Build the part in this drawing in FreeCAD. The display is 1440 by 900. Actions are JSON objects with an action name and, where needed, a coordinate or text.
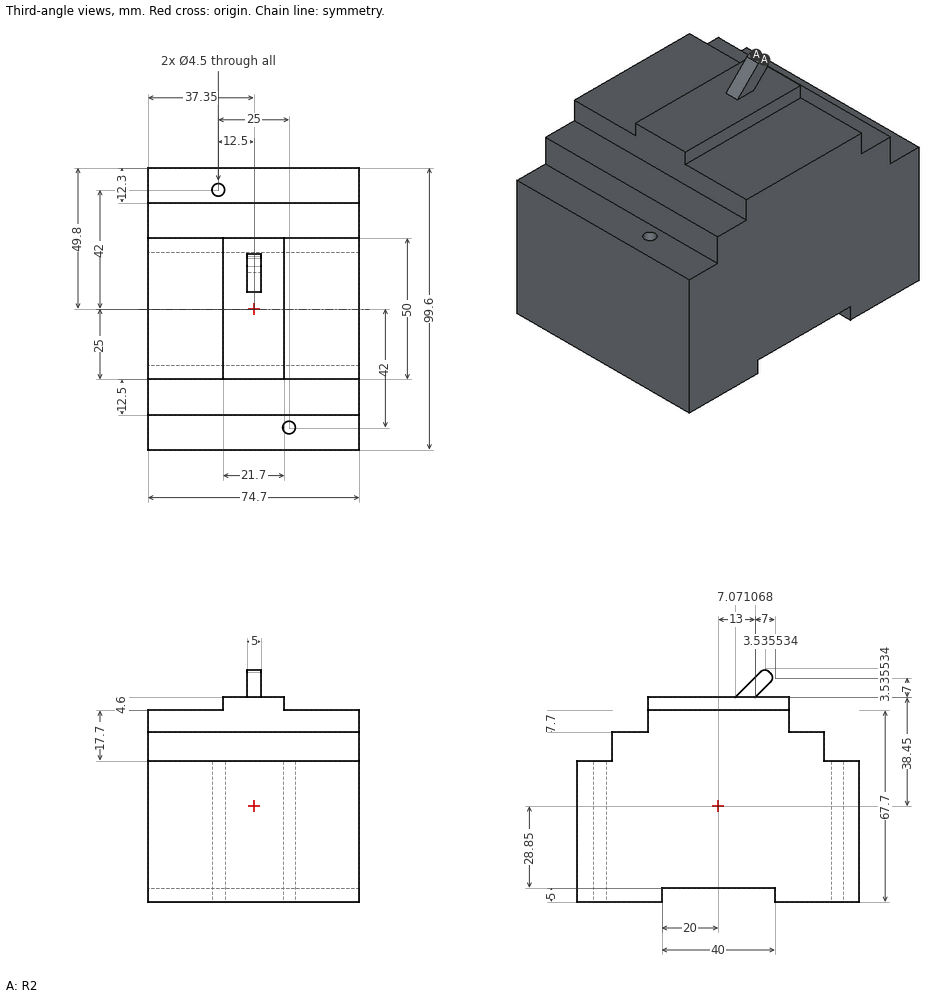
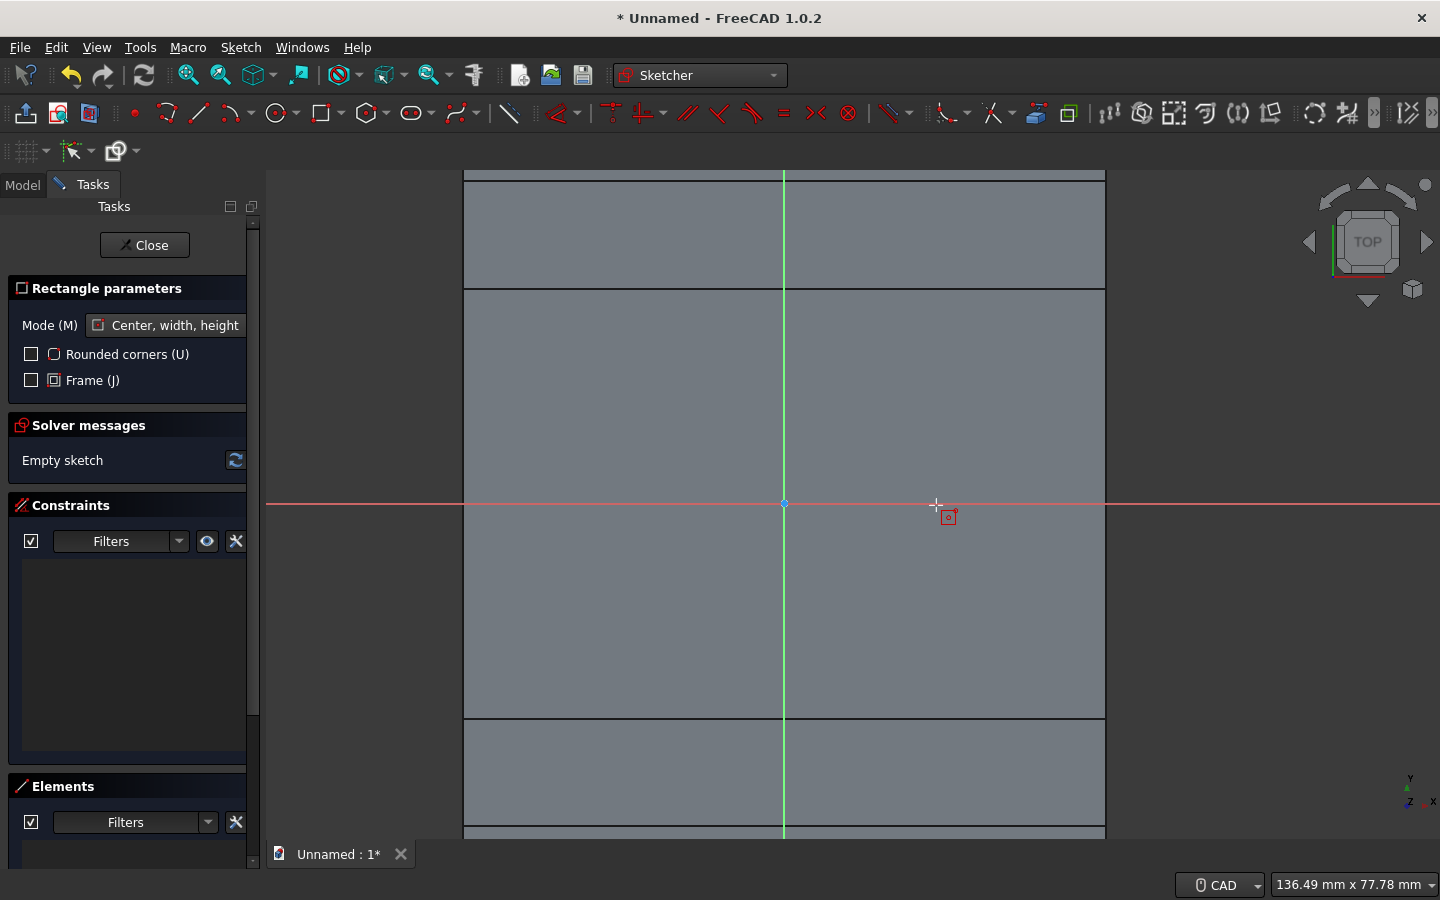
{"action": "left_click", "coordinate": [784, 504]}
{"action": "left_click", "coordinate": [878, 289]}
{"action": "key", "text": "Escape"}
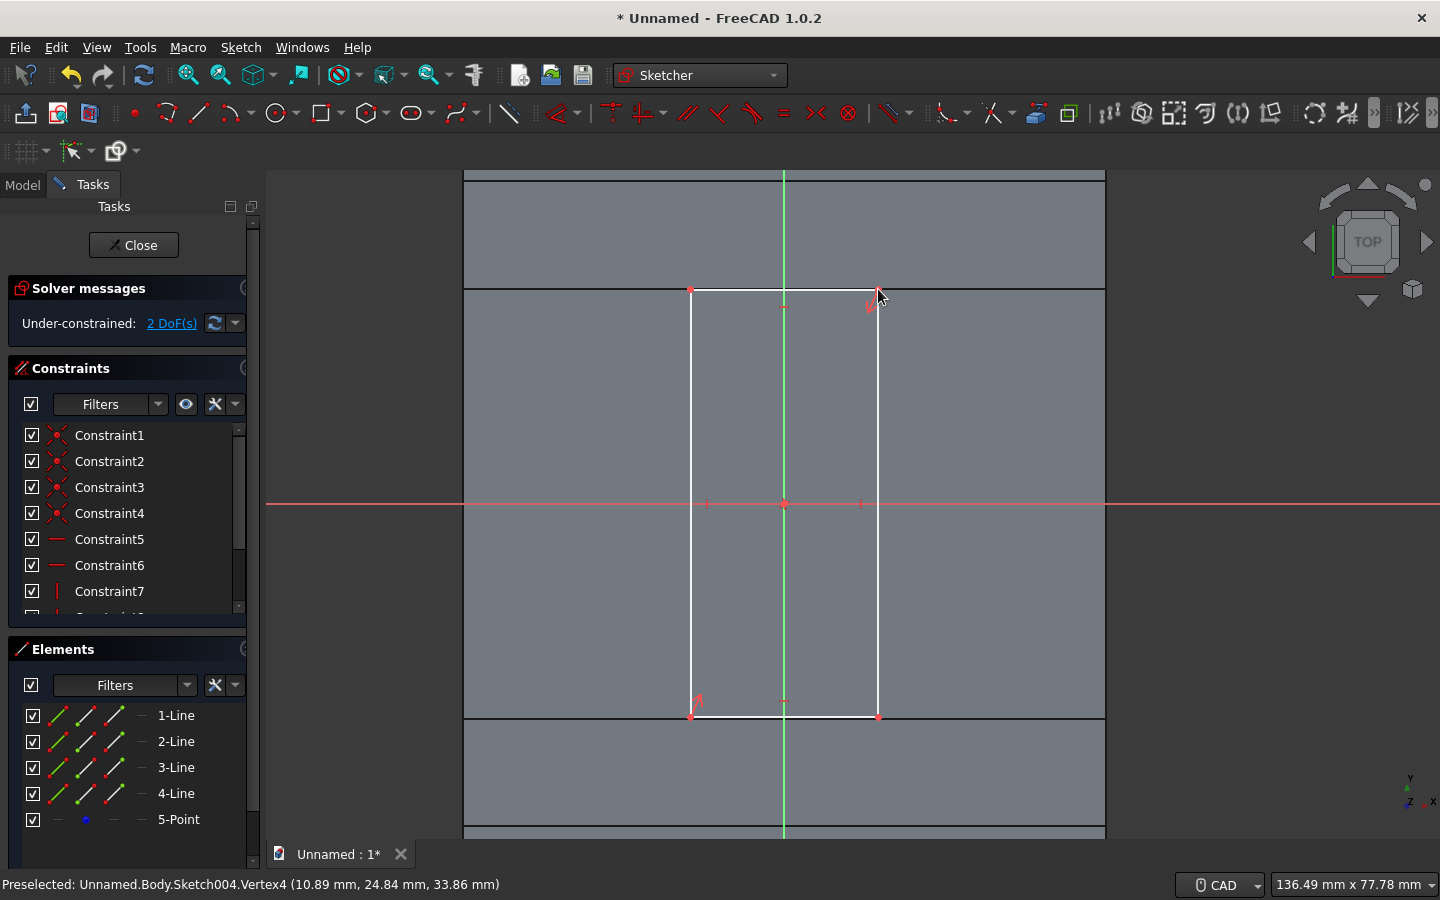
{"action": "left_click", "coordinate": [556, 114]}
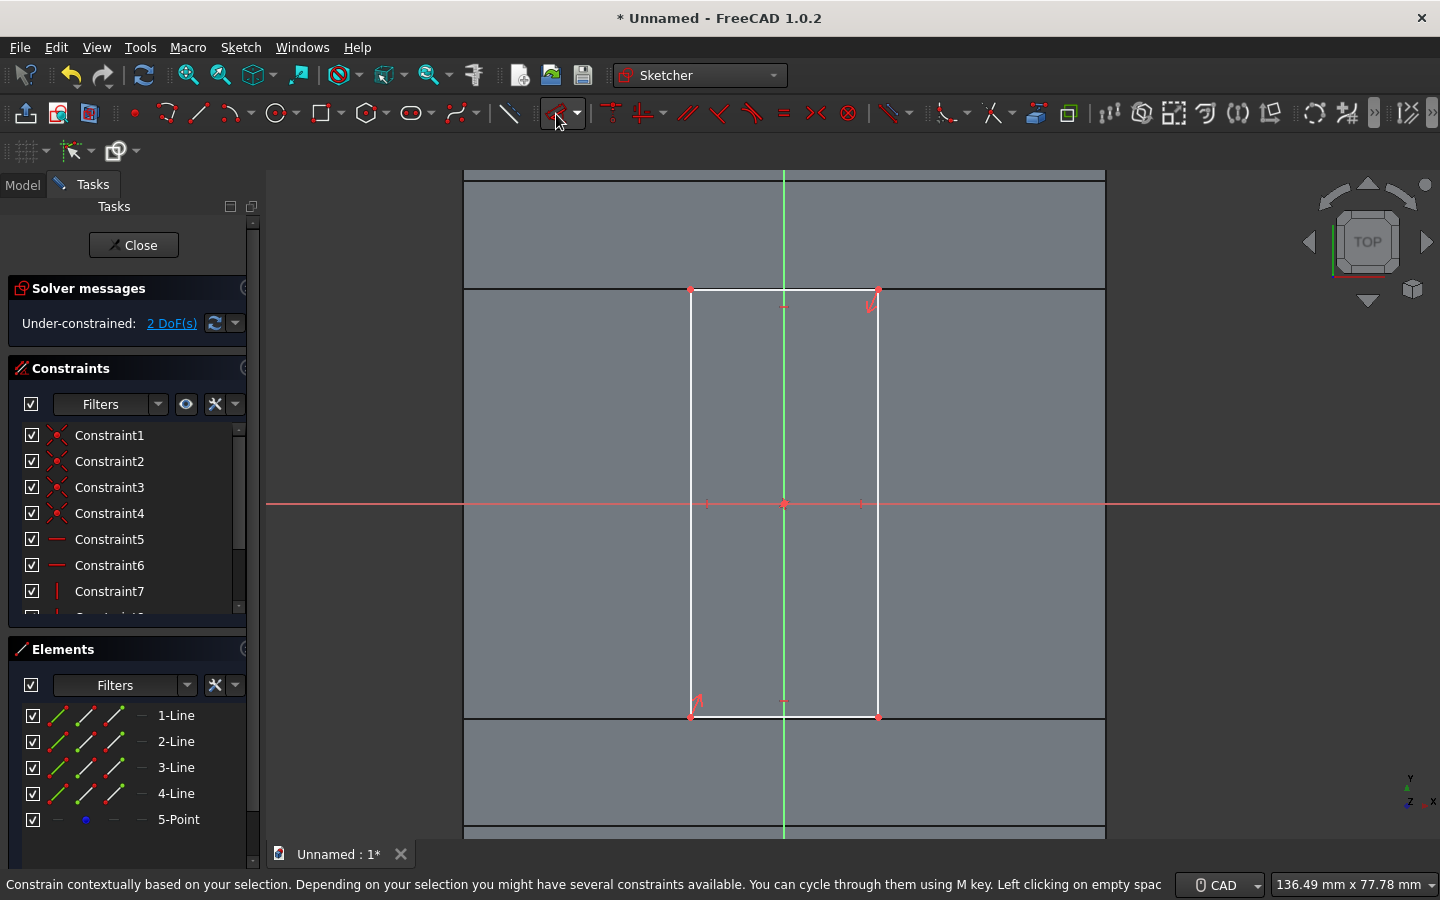
{"action": "left_click", "coordinate": [878, 589]}
{"action": "left_click", "coordinate": [912, 405]}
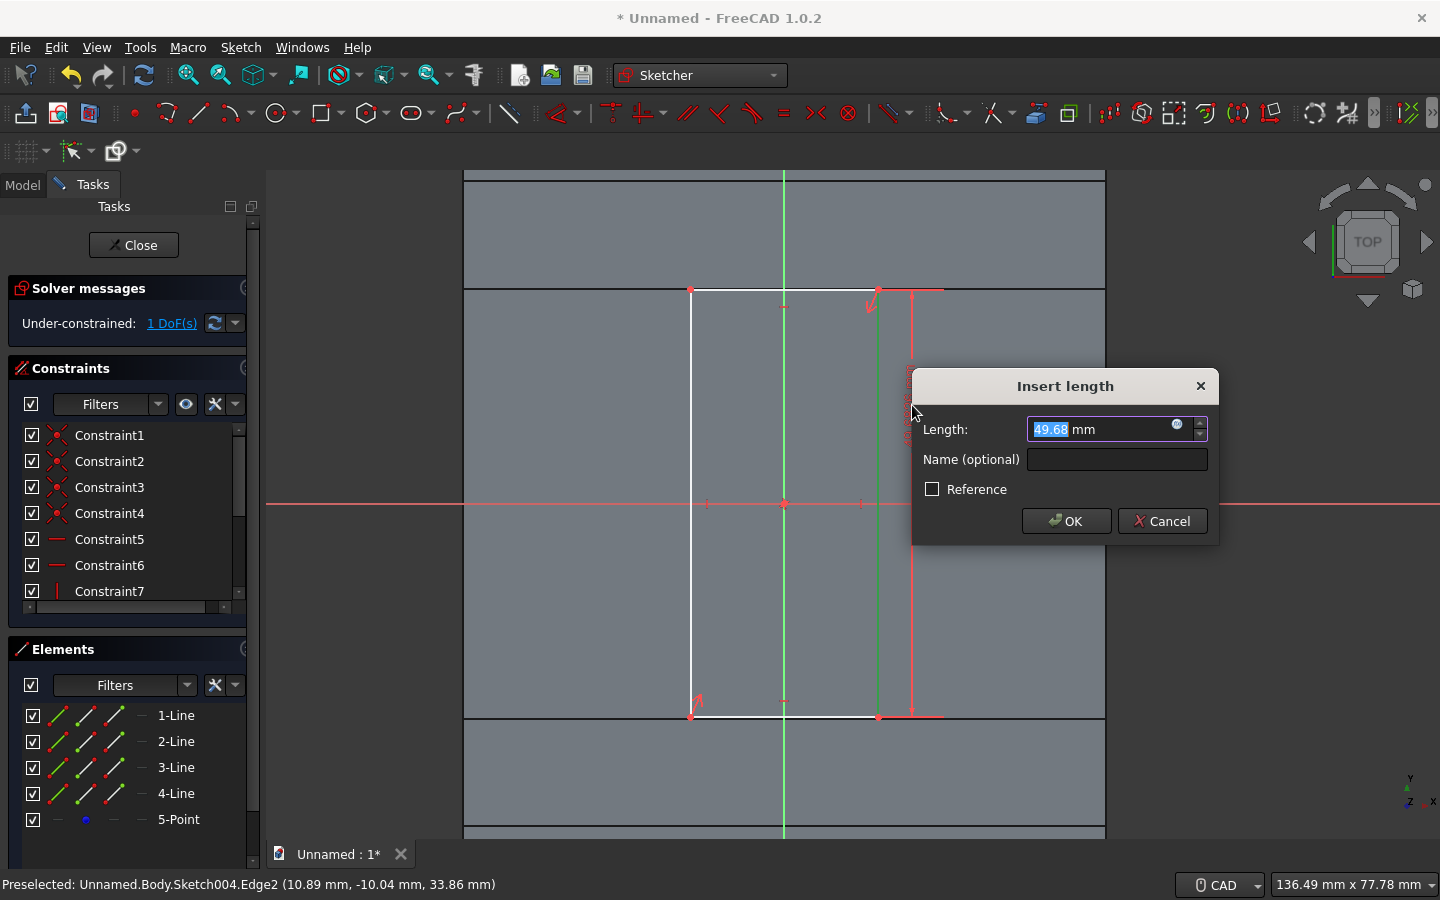
{"action": "type", "text": "50"}
{"action": "key", "text": "Return"}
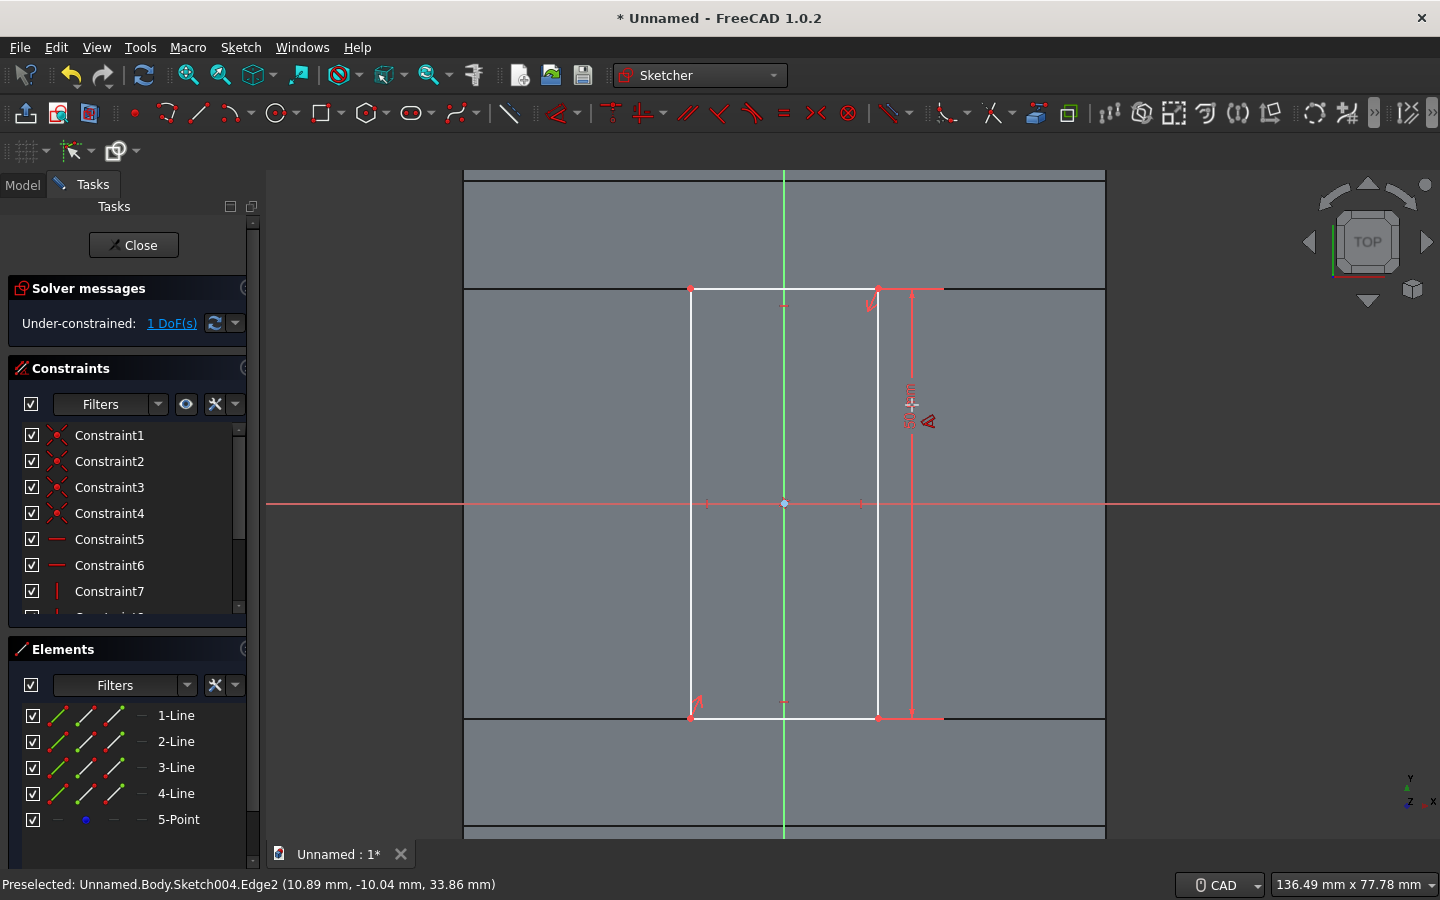
{"action": "left_click", "coordinate": [747, 719]}
{"action": "left_click", "coordinate": [741, 753]}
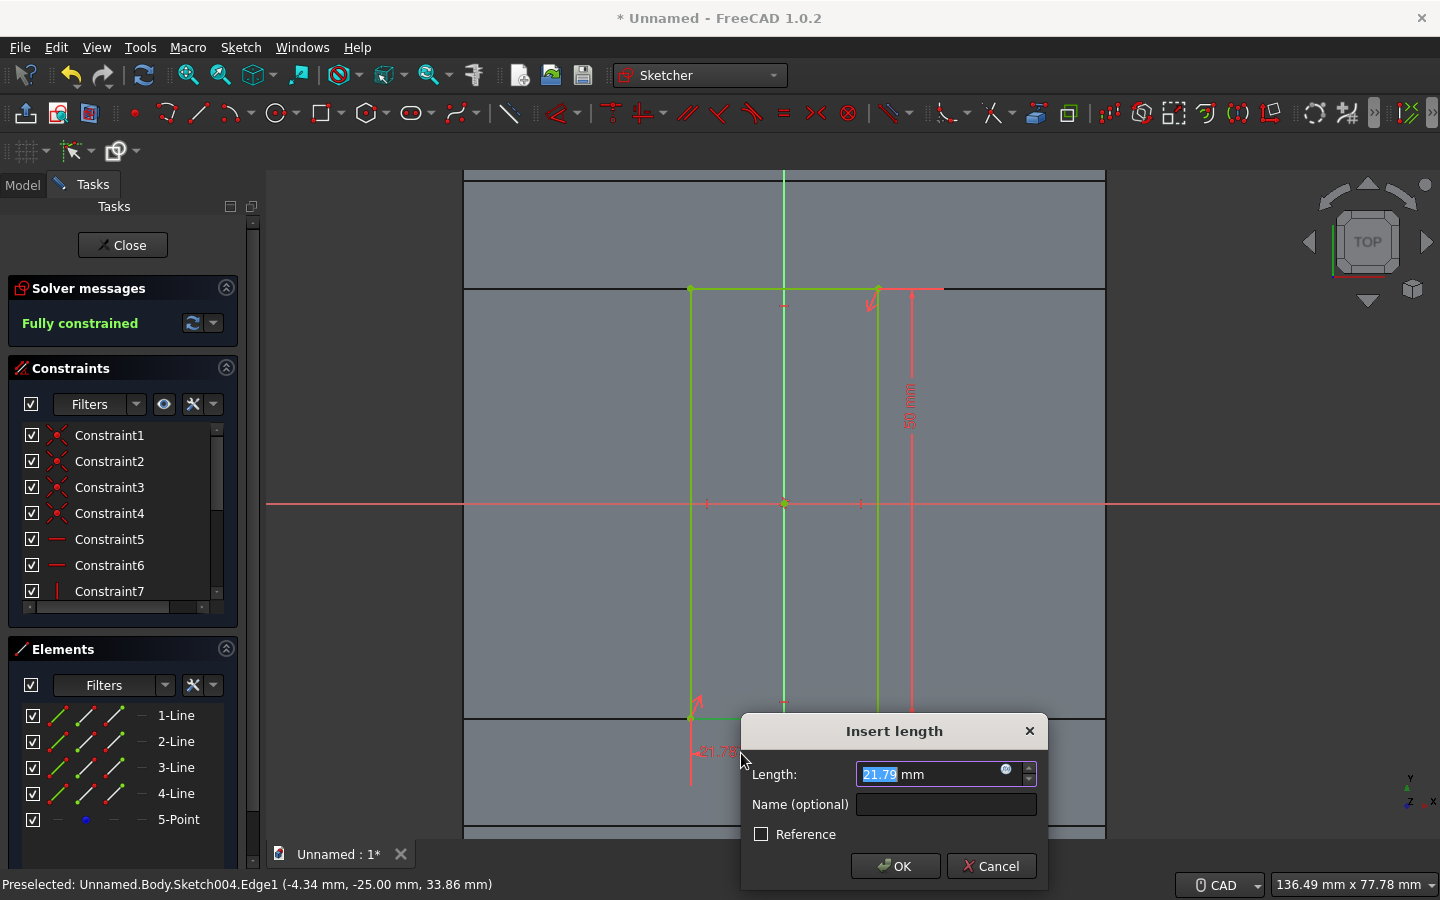
{"action": "type", "text": "21.7"}
{"action": "key", "text": "Return"}
{"action": "key", "text": "Escape"}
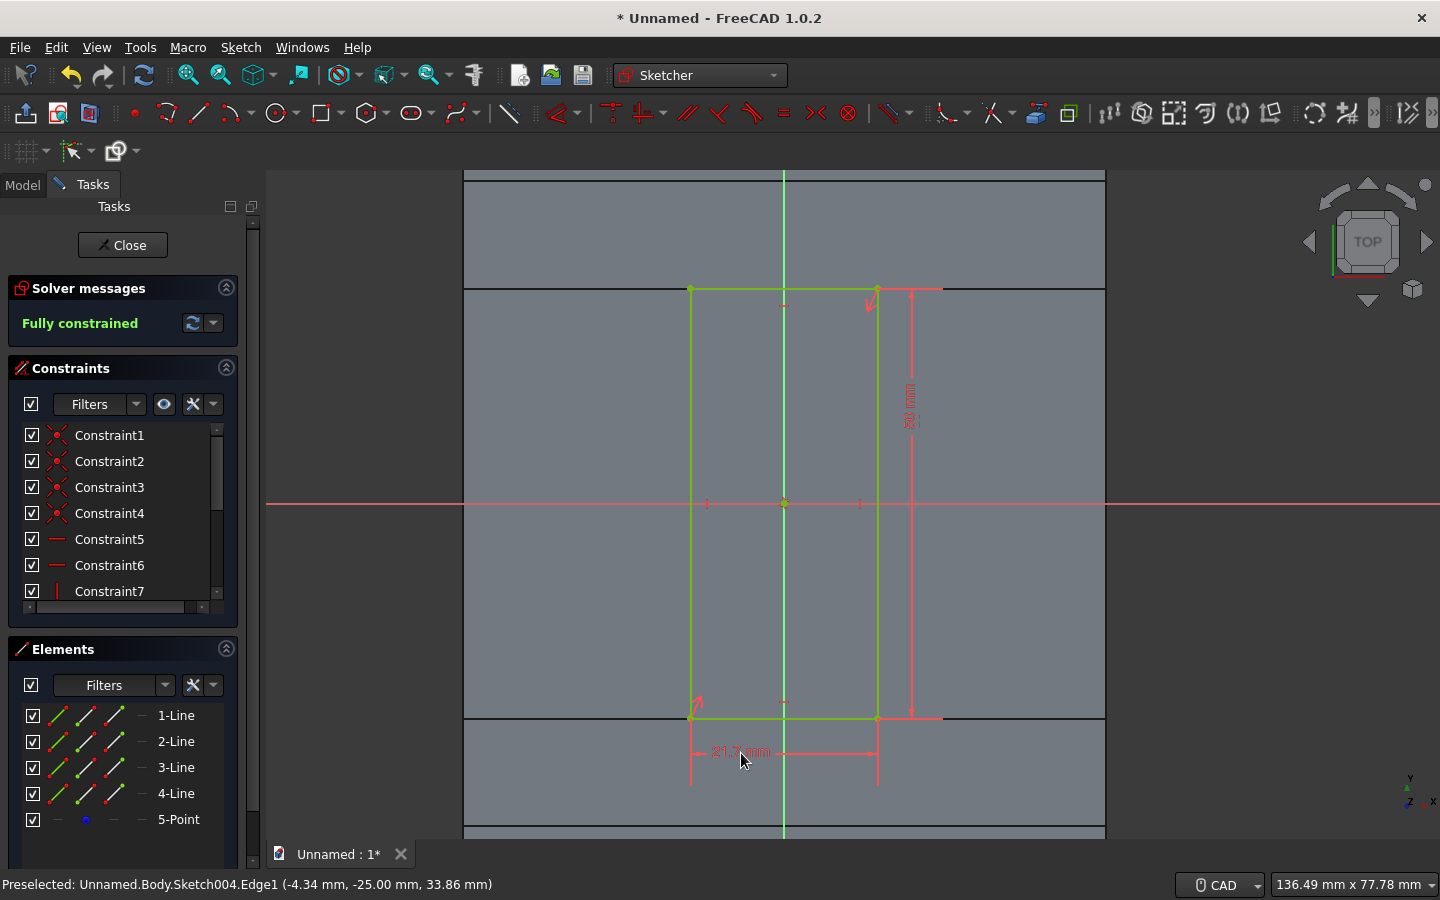
{"action": "left_click", "coordinate": [123, 245]}